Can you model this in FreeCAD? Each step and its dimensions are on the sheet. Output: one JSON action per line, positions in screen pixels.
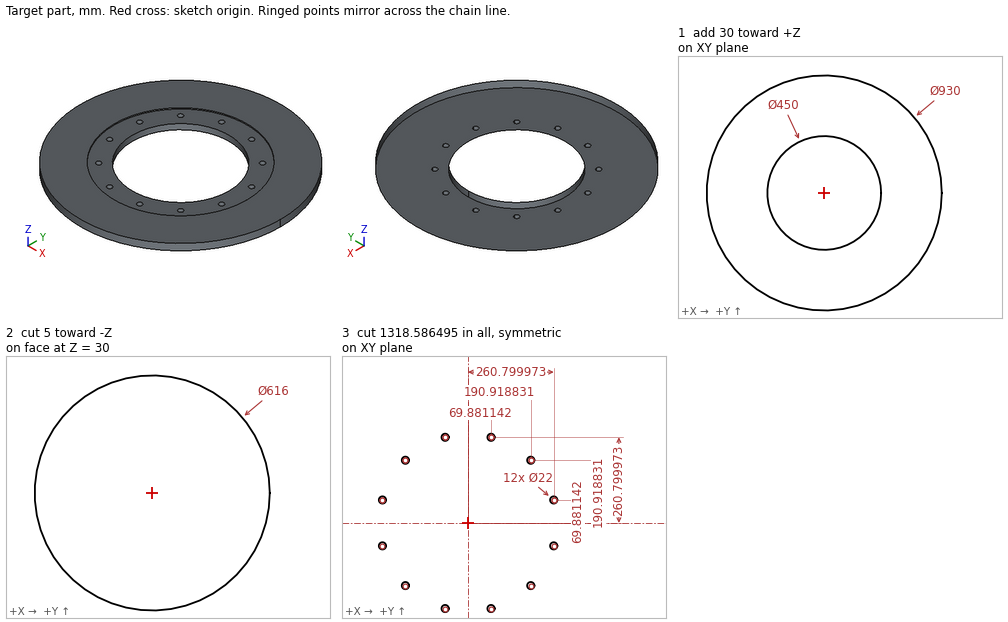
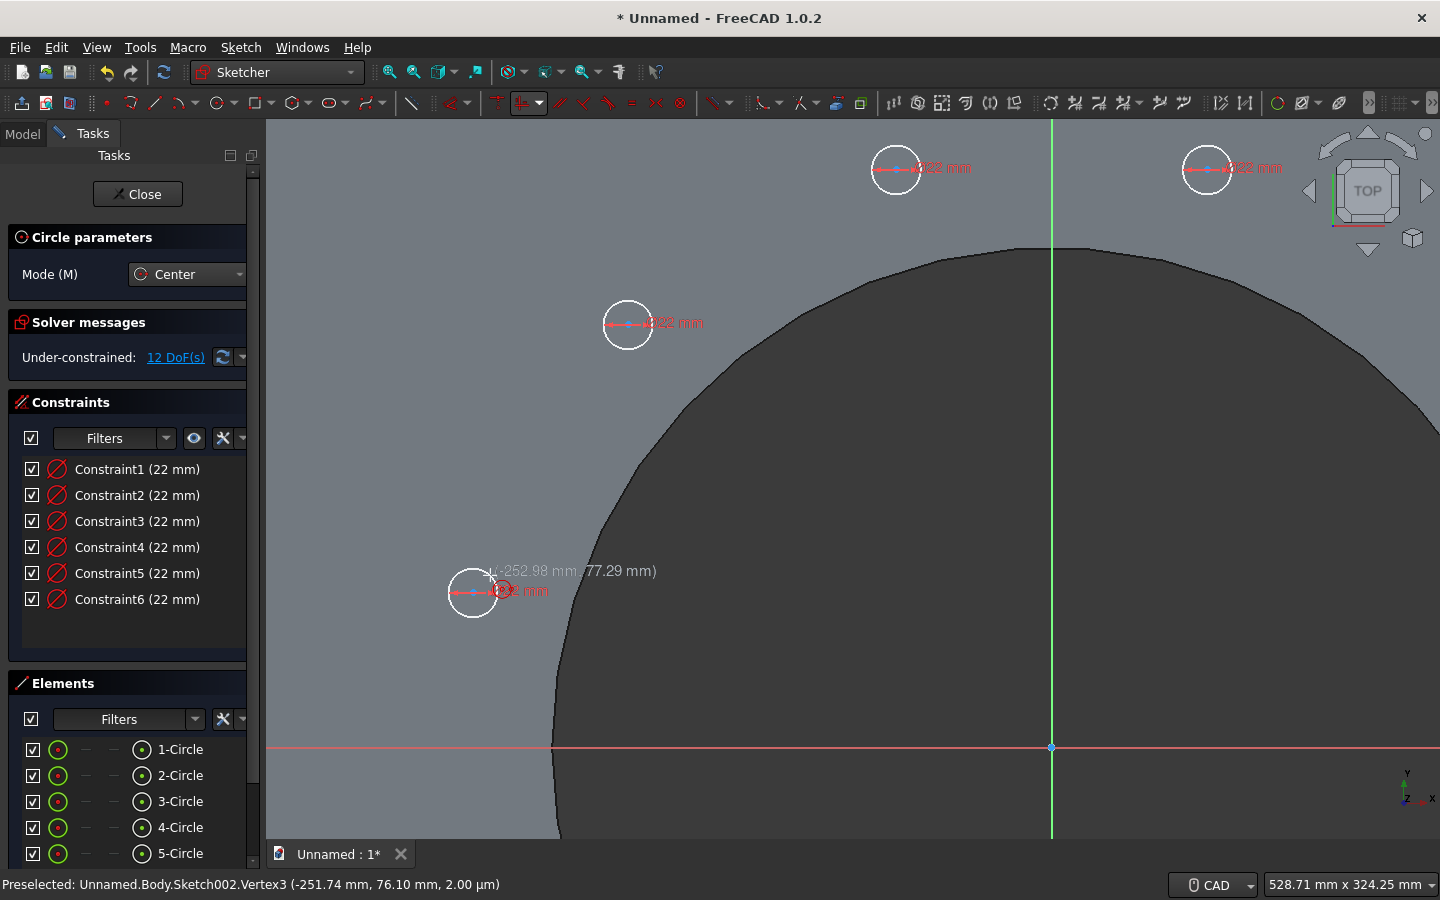
{"action": "scroll", "coordinate": [629, 323], "scroll_direction": "down", "scroll_amount": 5}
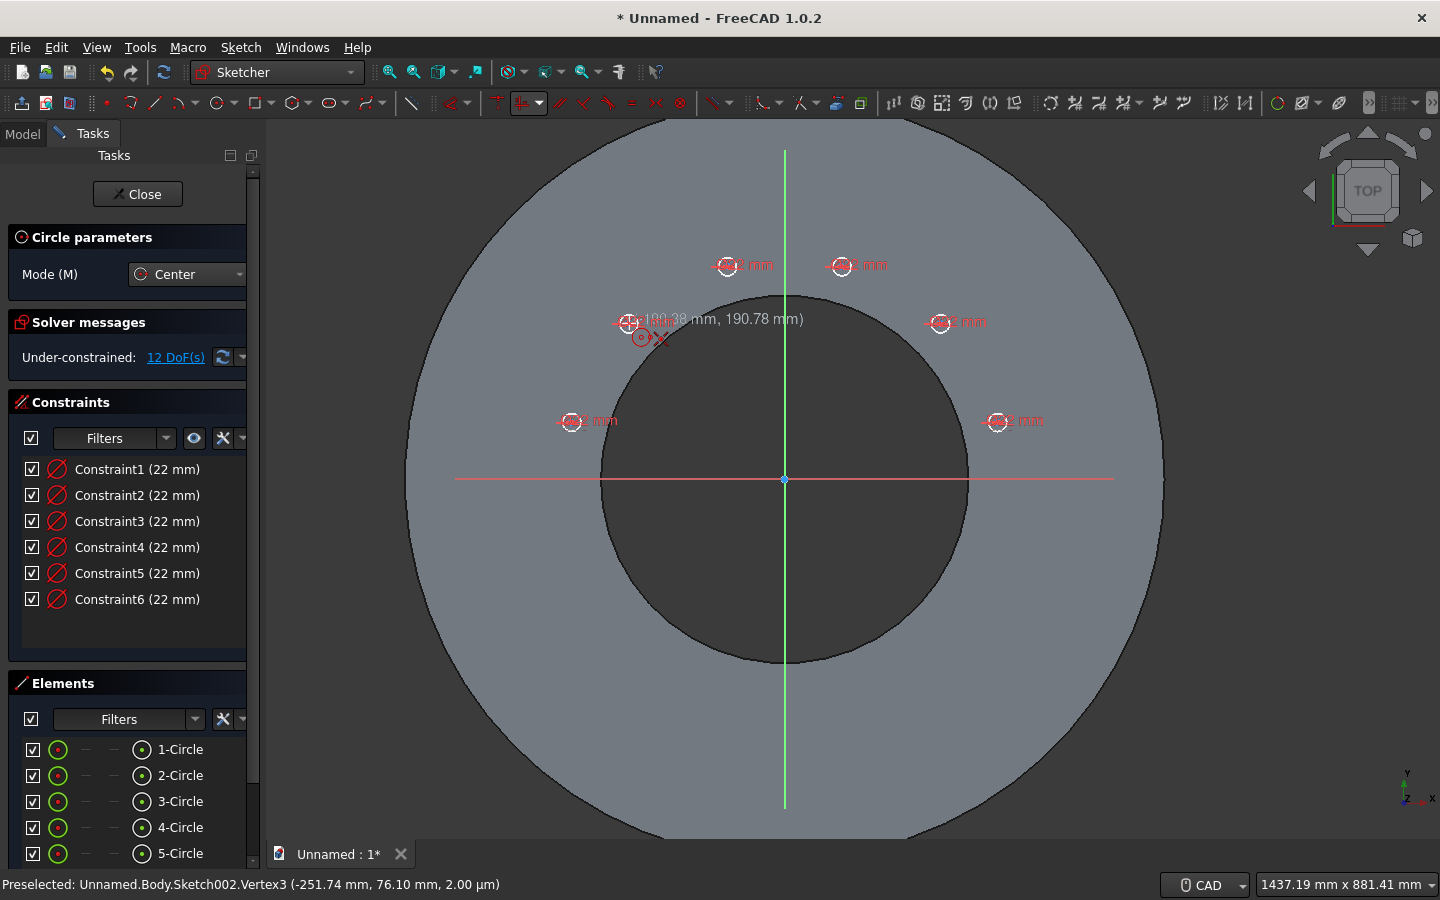
{"action": "scroll", "coordinate": [572, 536], "scroll_direction": "up", "scroll_amount": 5}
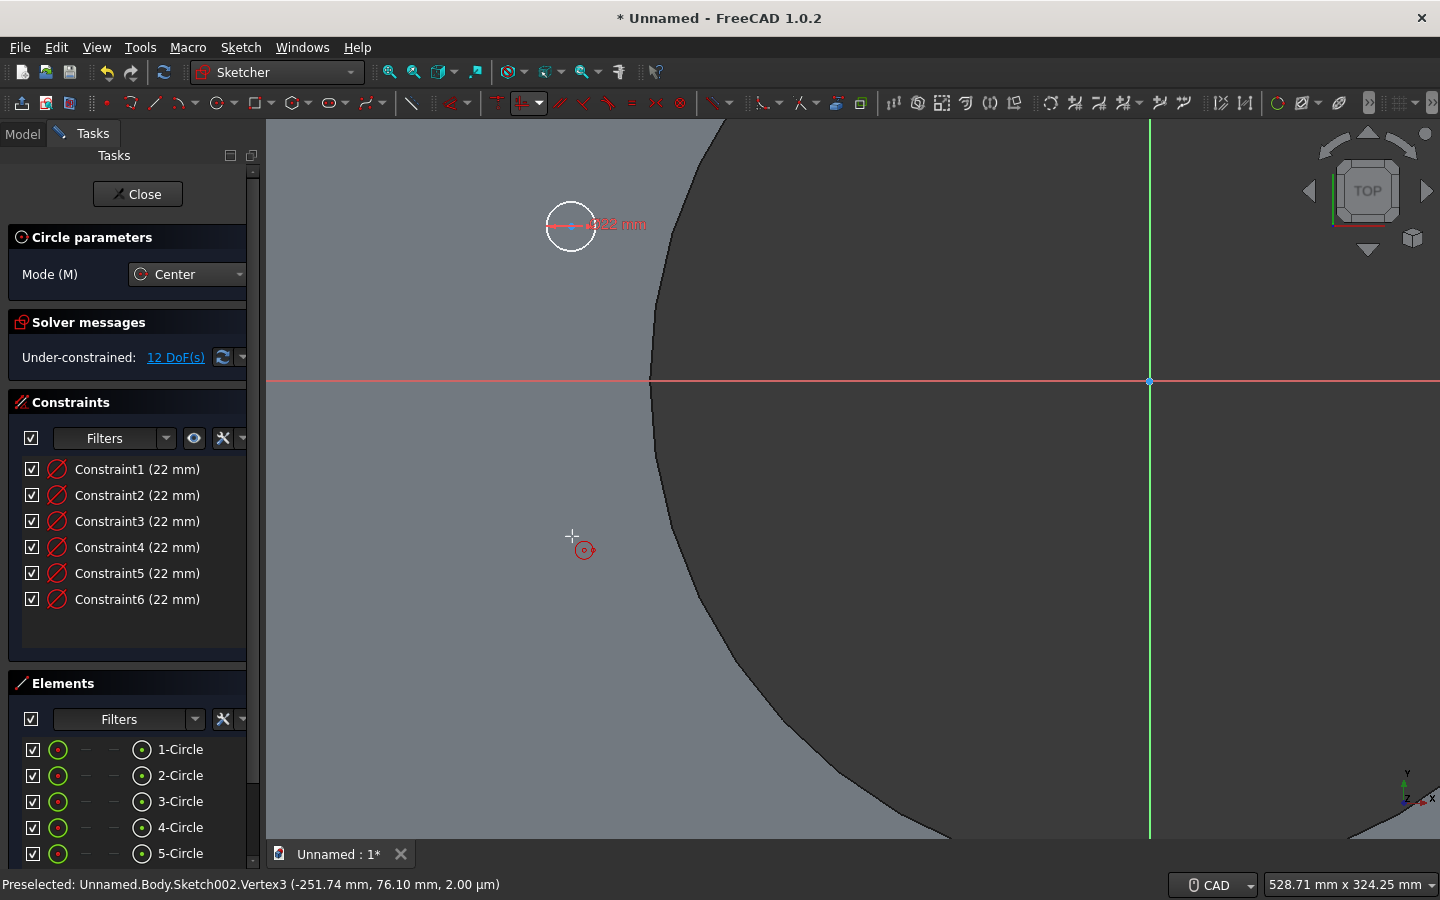
{"action": "left_click", "coordinate": [571, 536]}
{"action": "mouse_move", "coordinate": [588, 519]}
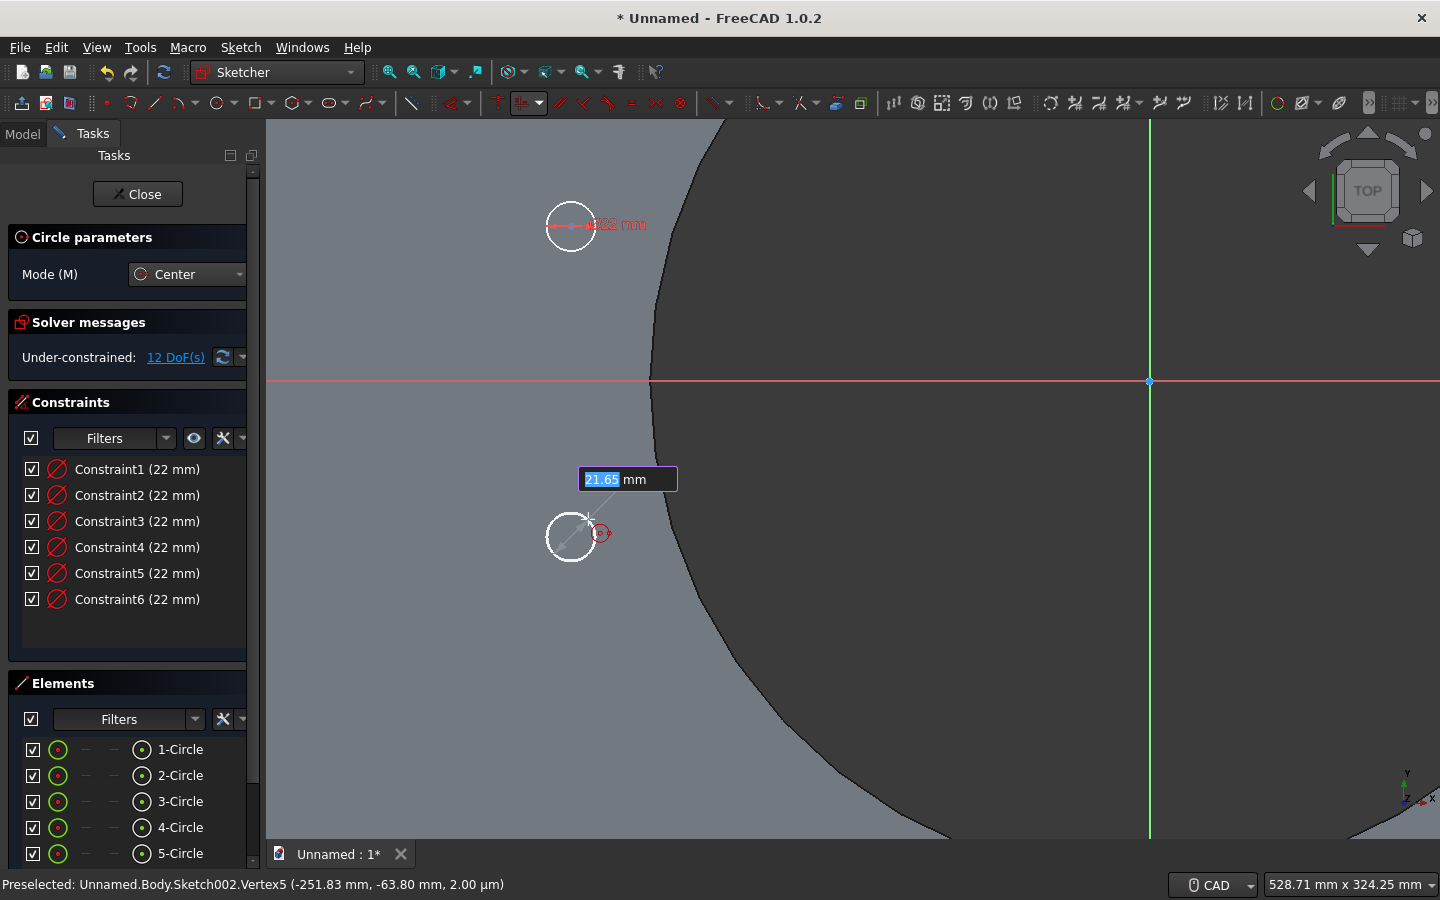
{"action": "type", "text": "22"}
{"action": "key", "text": "Return"}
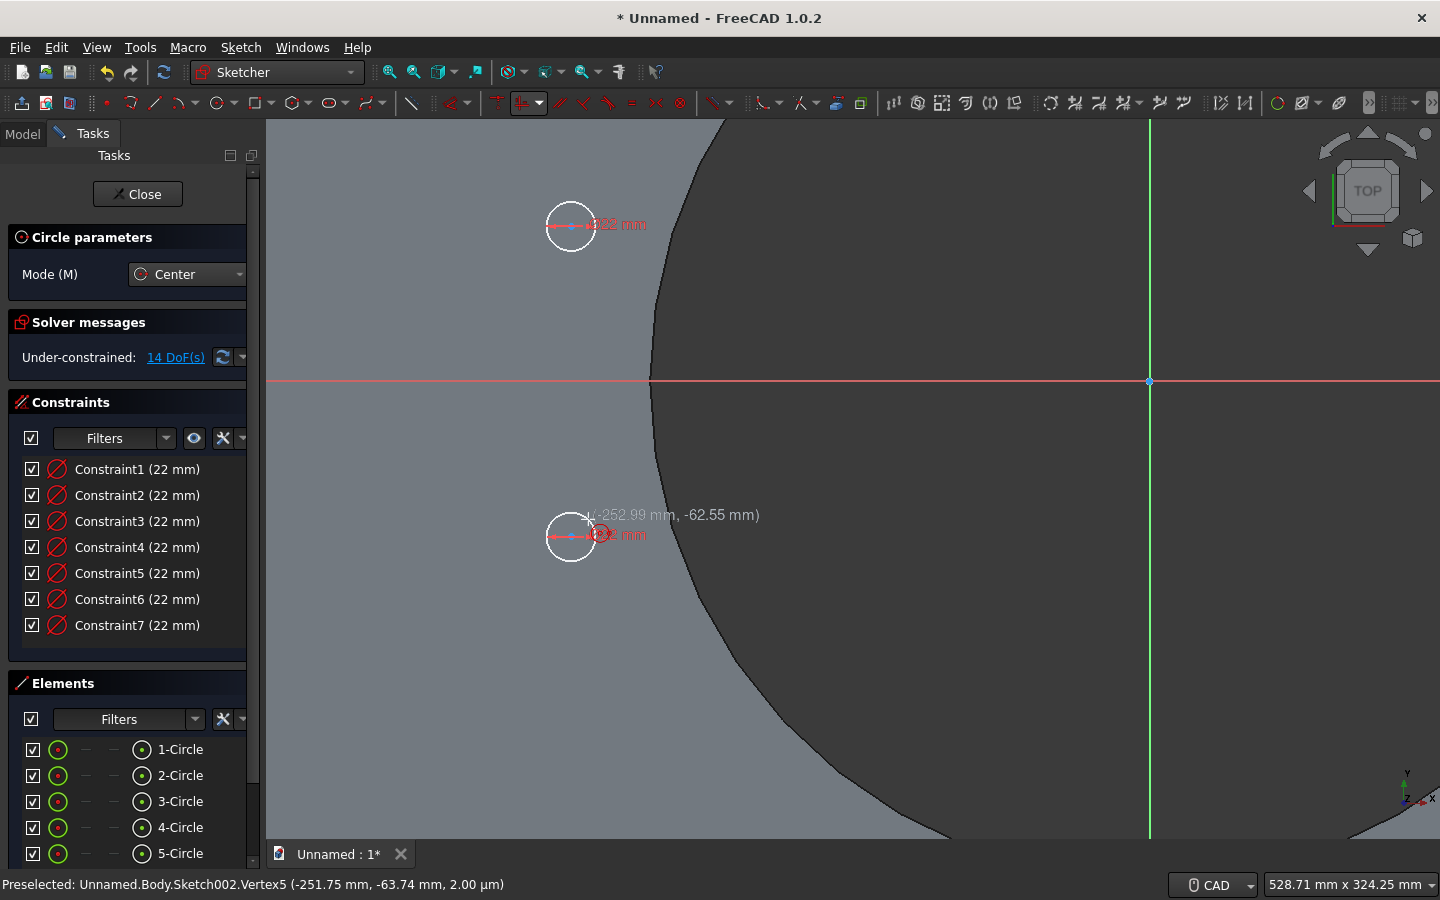
{"action": "left_click", "coordinate": [726, 805]}
{"action": "mouse_move", "coordinate": [743, 788]}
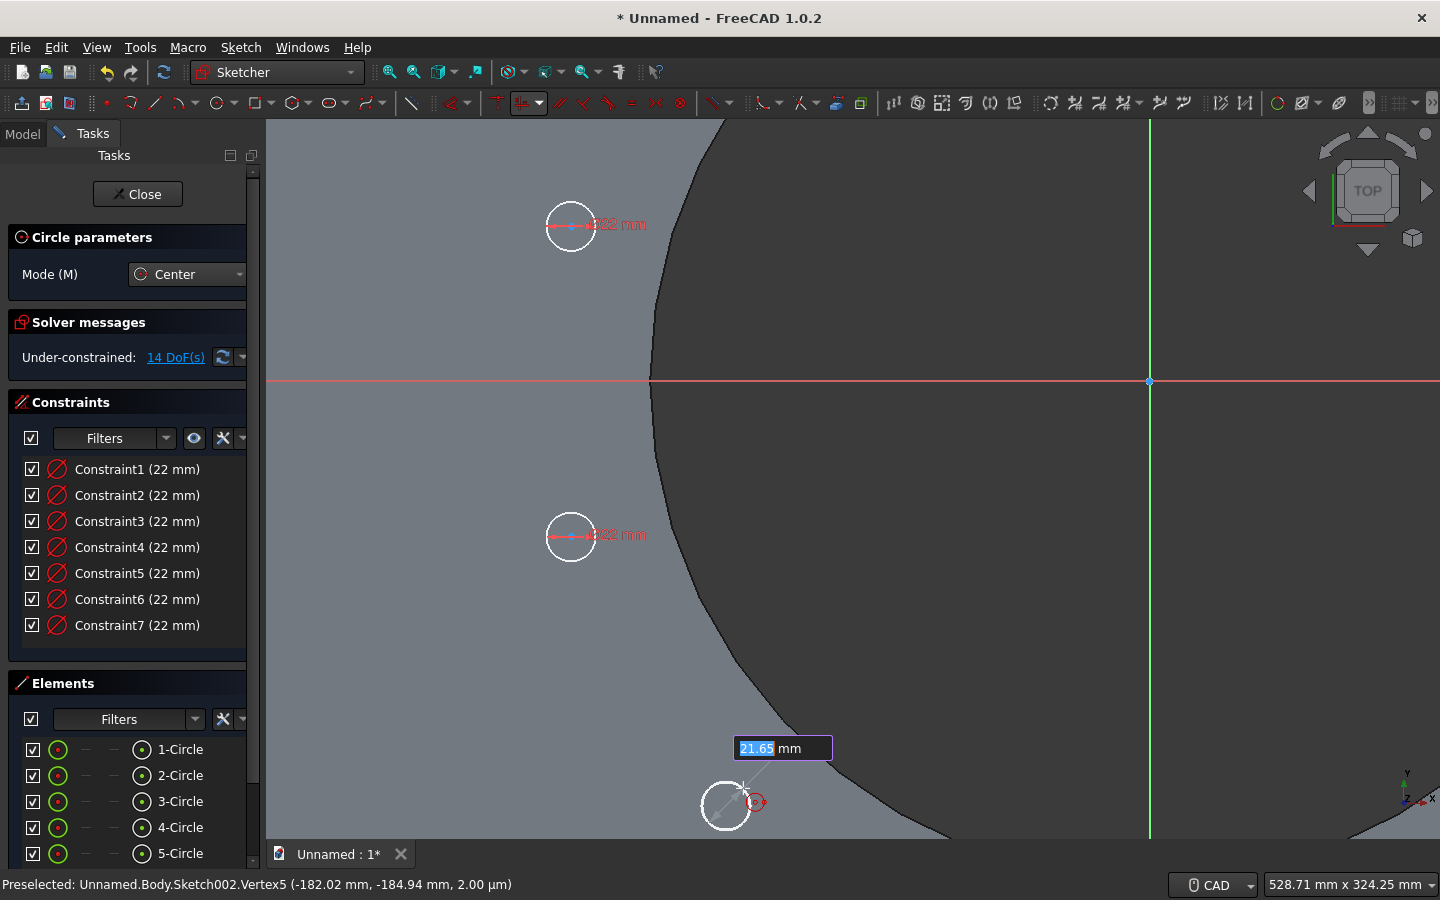
{"action": "type", "text": "22"}
{"action": "key", "text": "Return"}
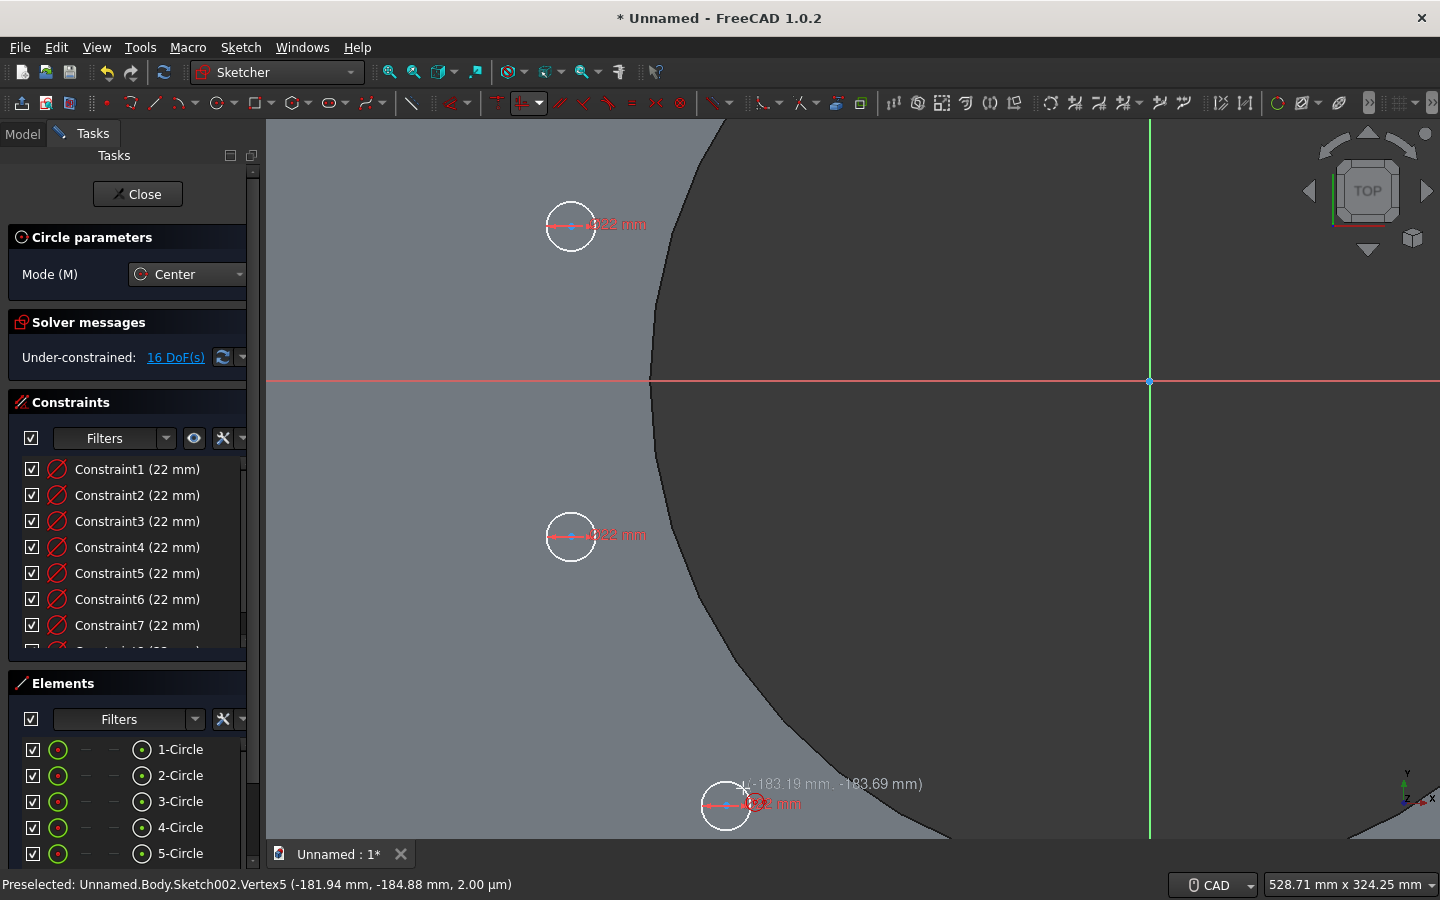
{"action": "scroll", "coordinate": [572, 536], "scroll_direction": "down", "scroll_amount": 5}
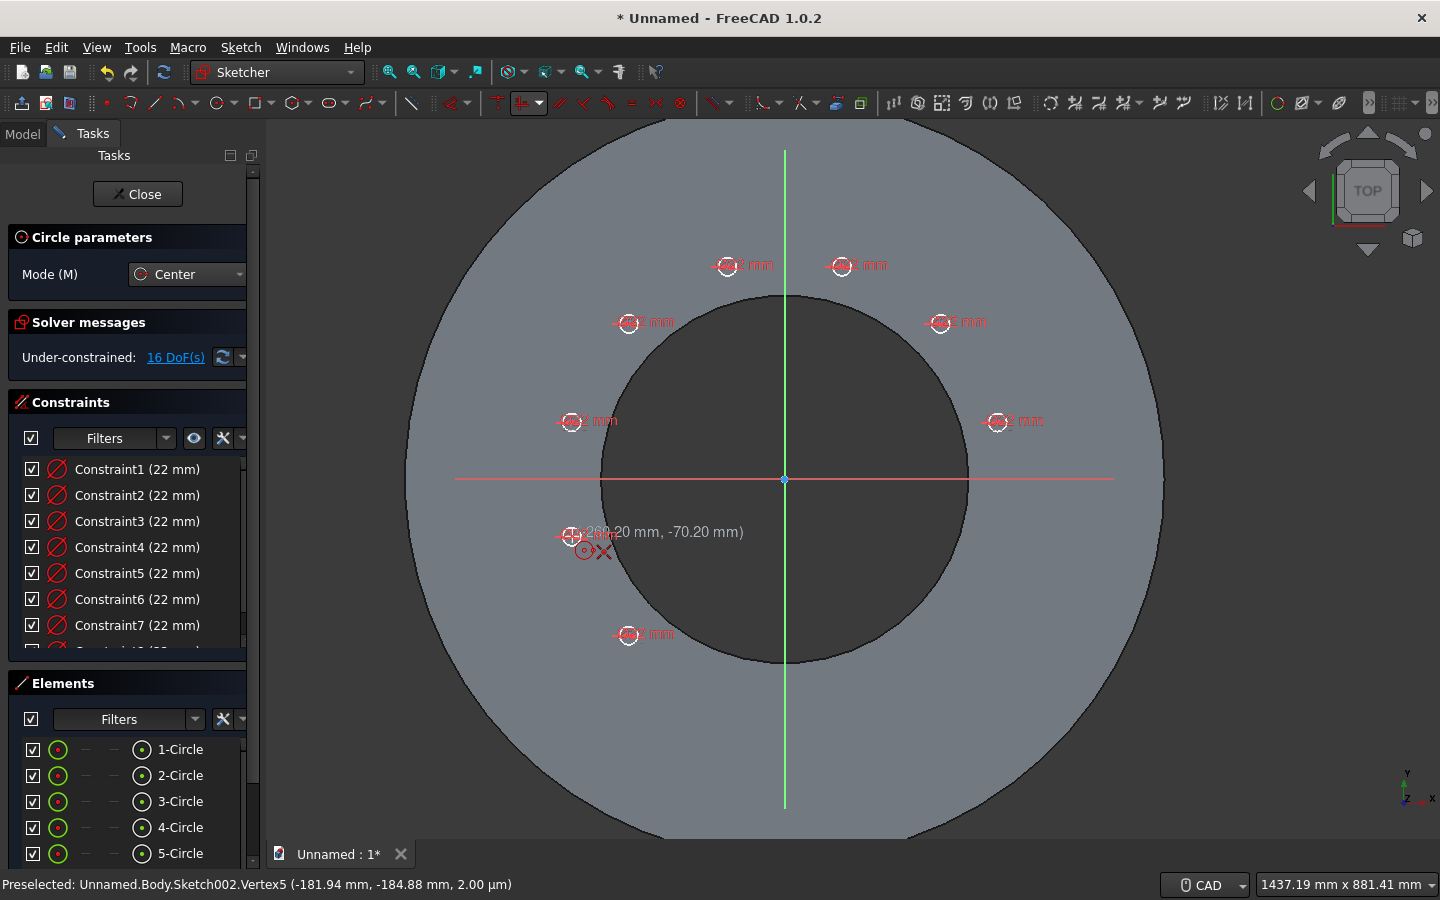
{"action": "scroll", "coordinate": [728, 692], "scroll_direction": "up", "scroll_amount": 5}